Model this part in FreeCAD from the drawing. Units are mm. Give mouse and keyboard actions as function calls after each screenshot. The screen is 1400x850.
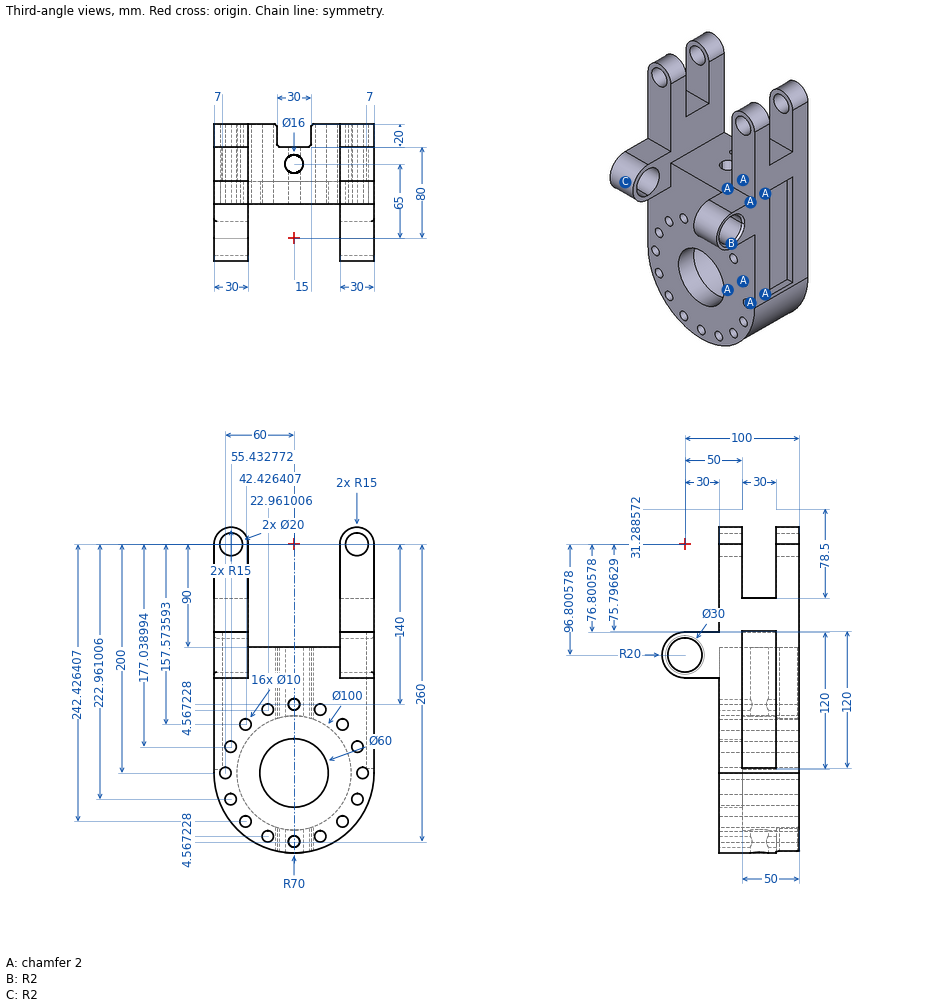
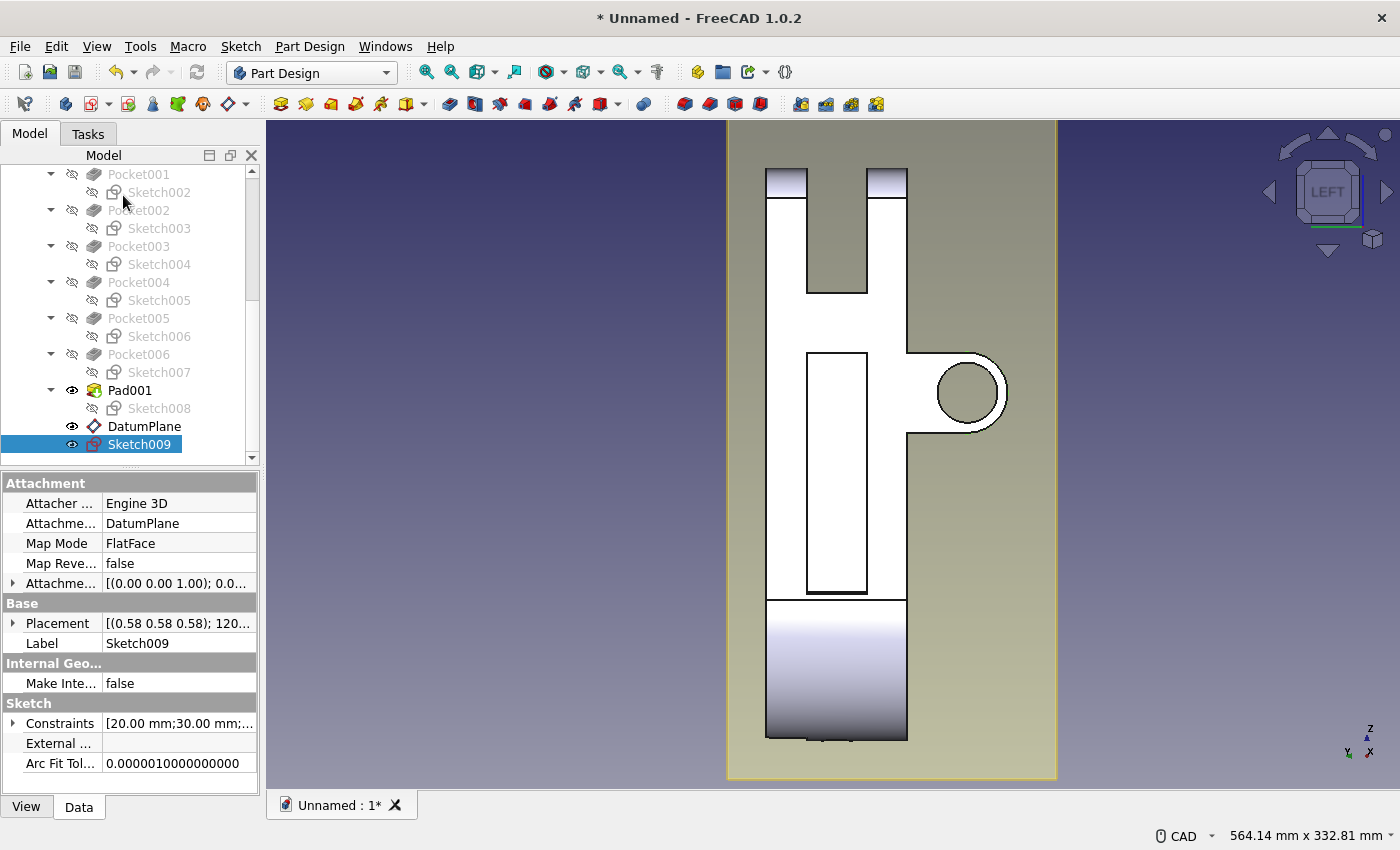
click(281, 104)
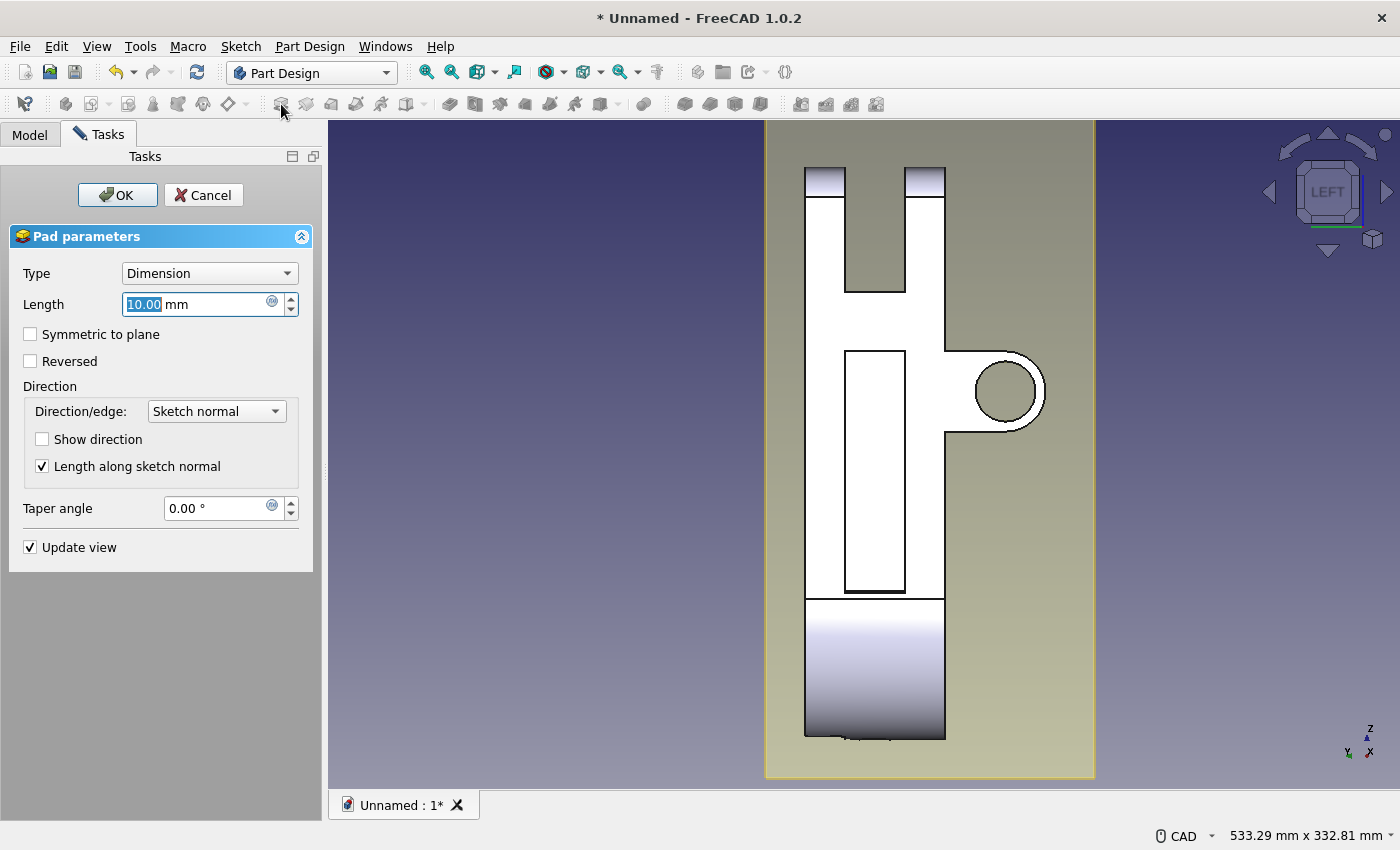
text(30)
key(Tab)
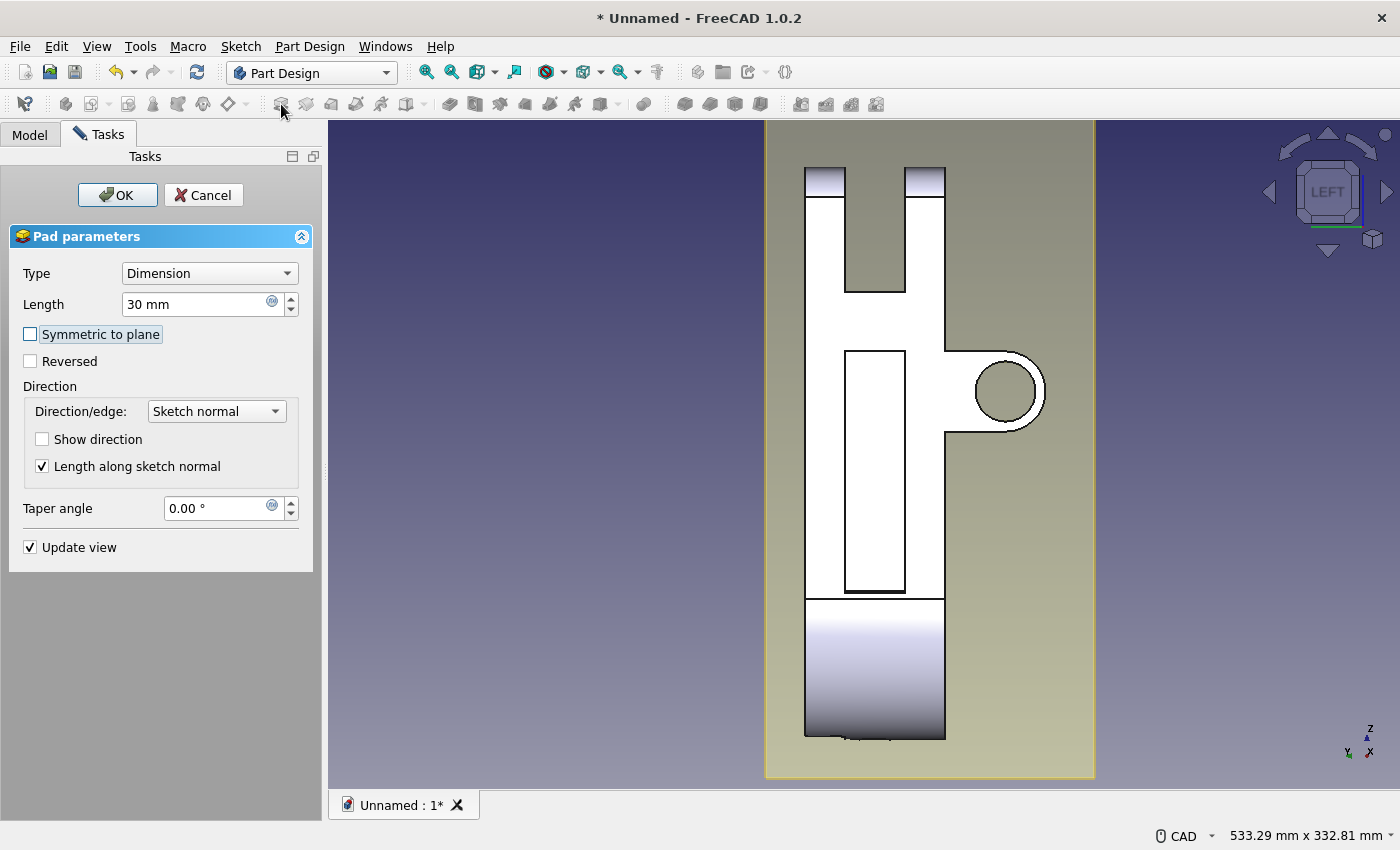
click(118, 195)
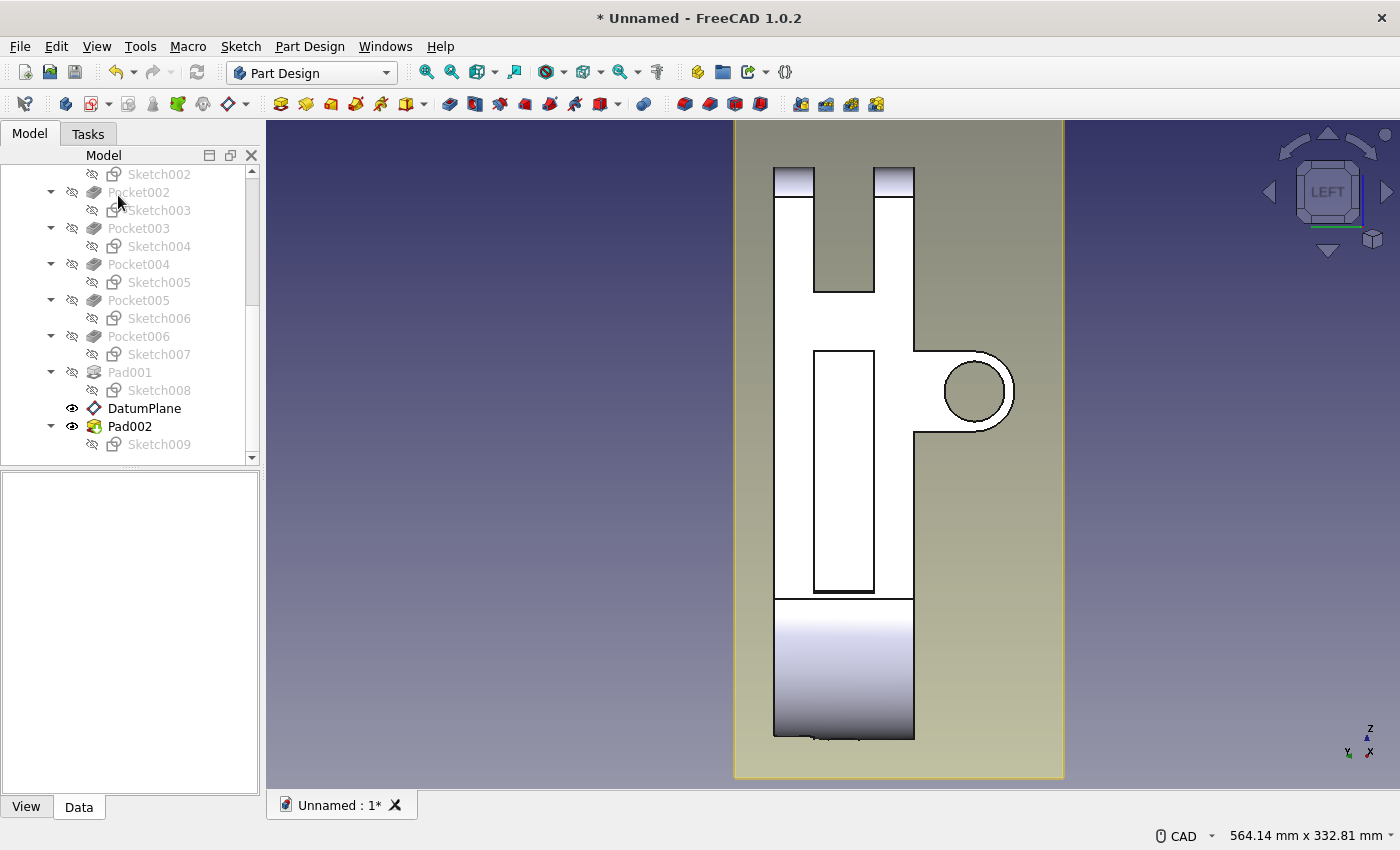
click(117, 408)
key(space)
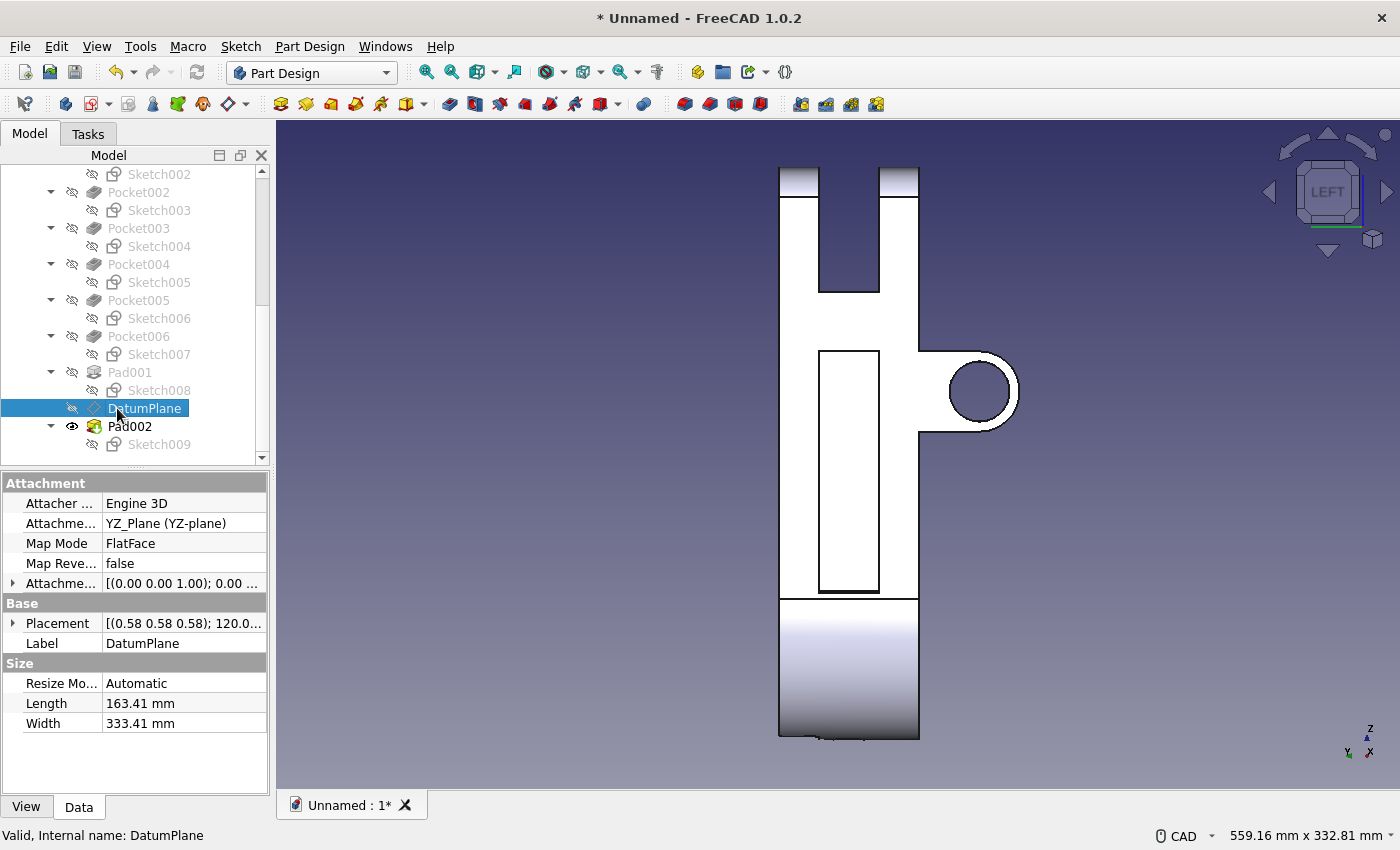
key(0)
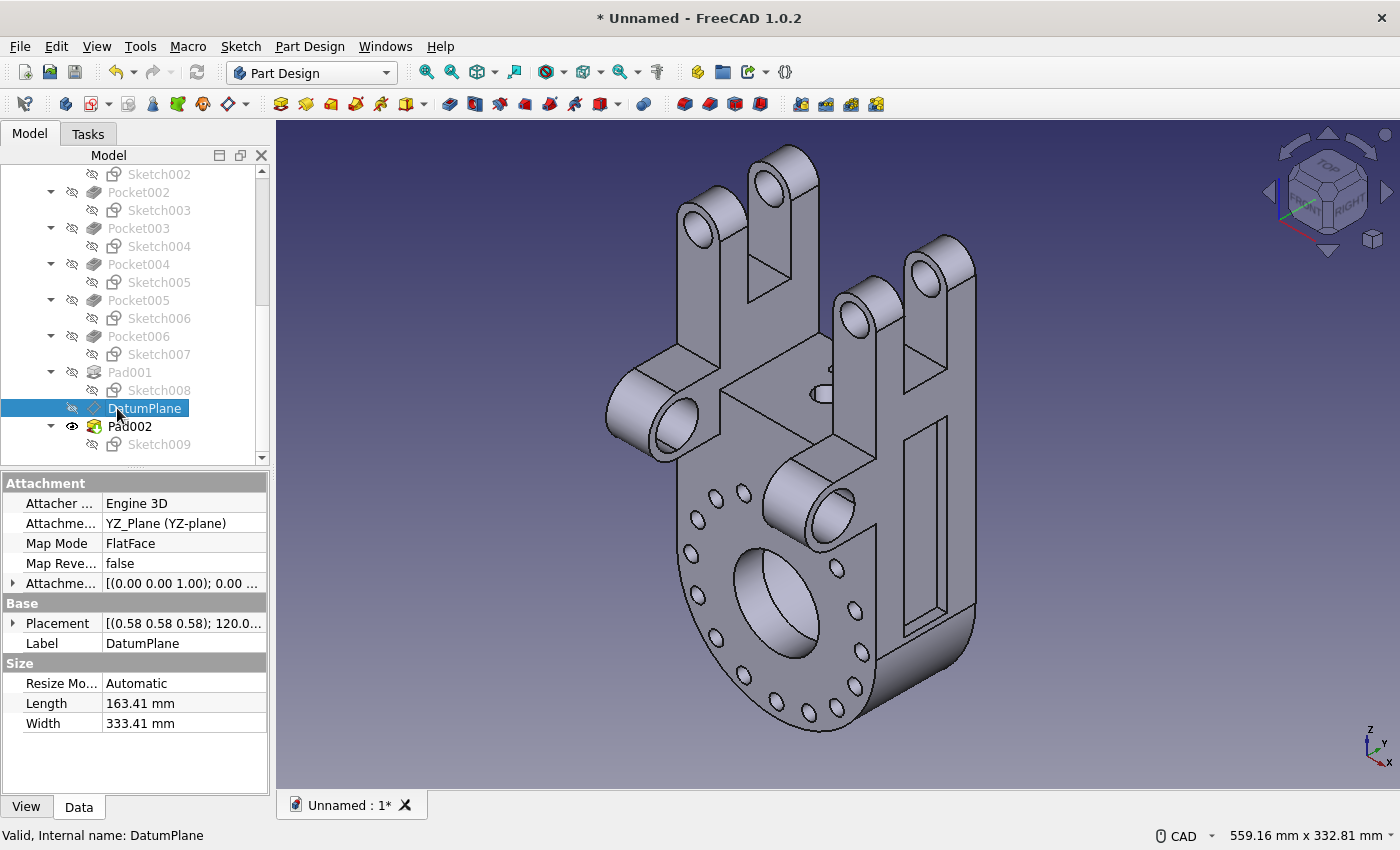
click(427, 72)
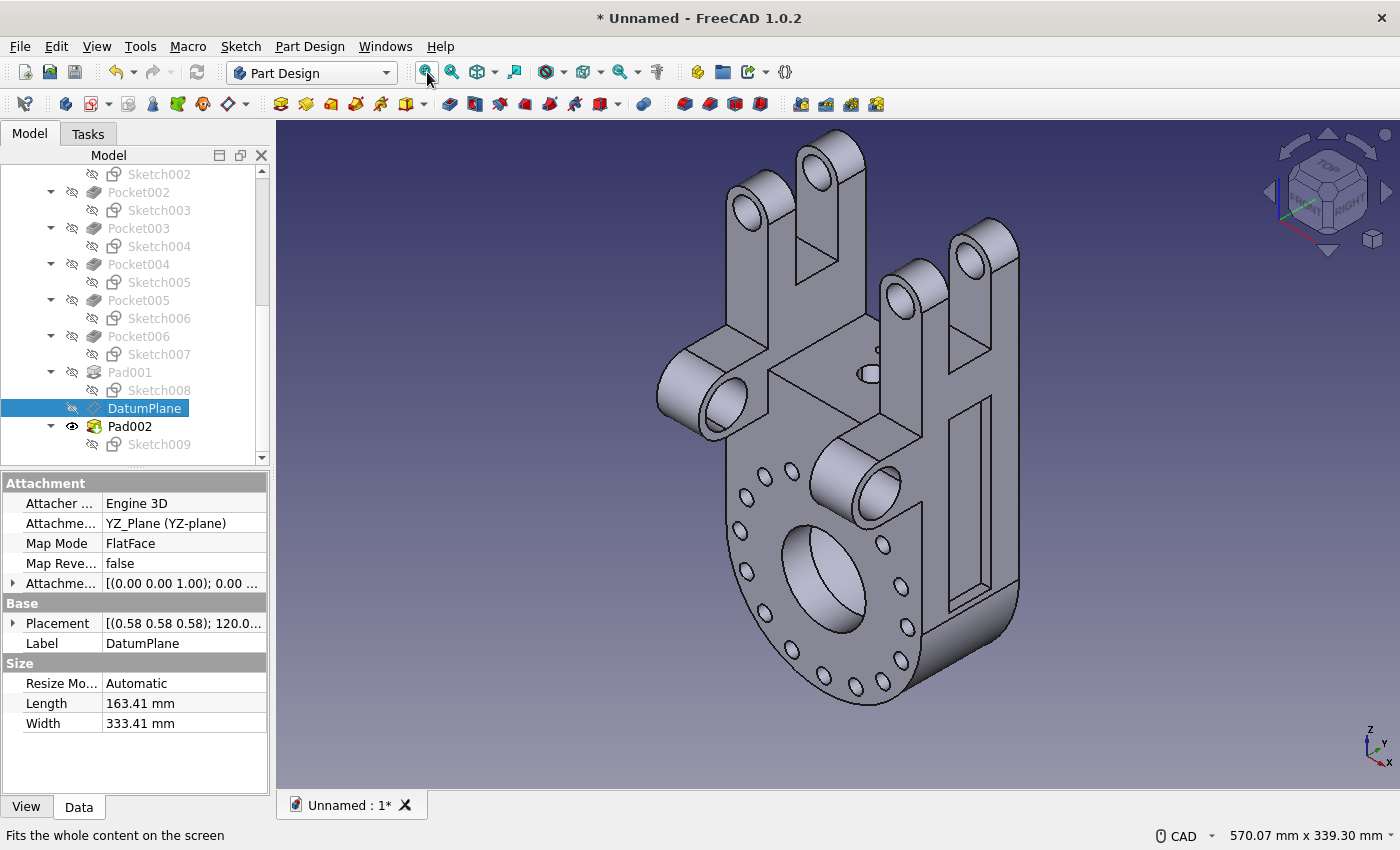
click(873, 519)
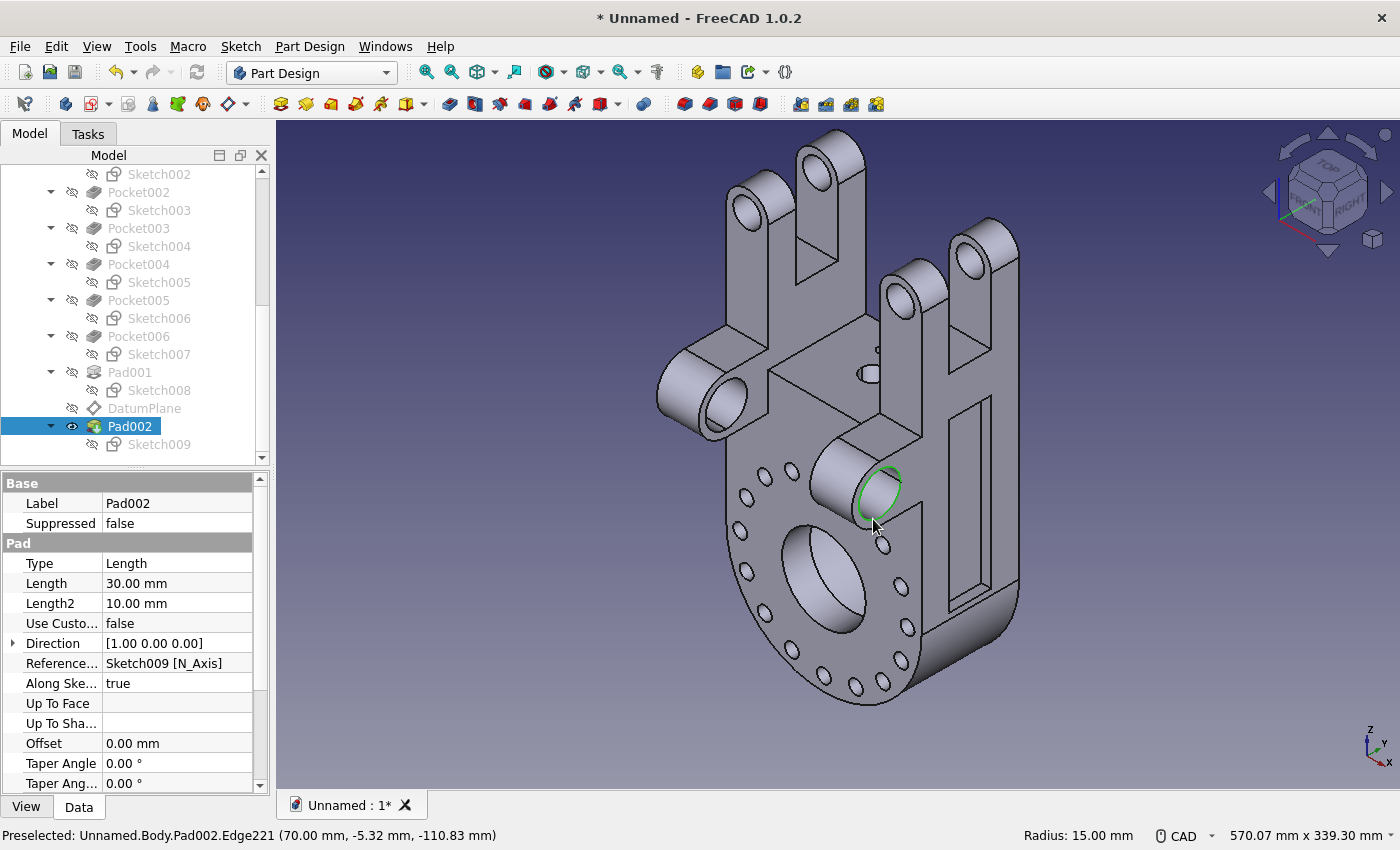
click(685, 104)